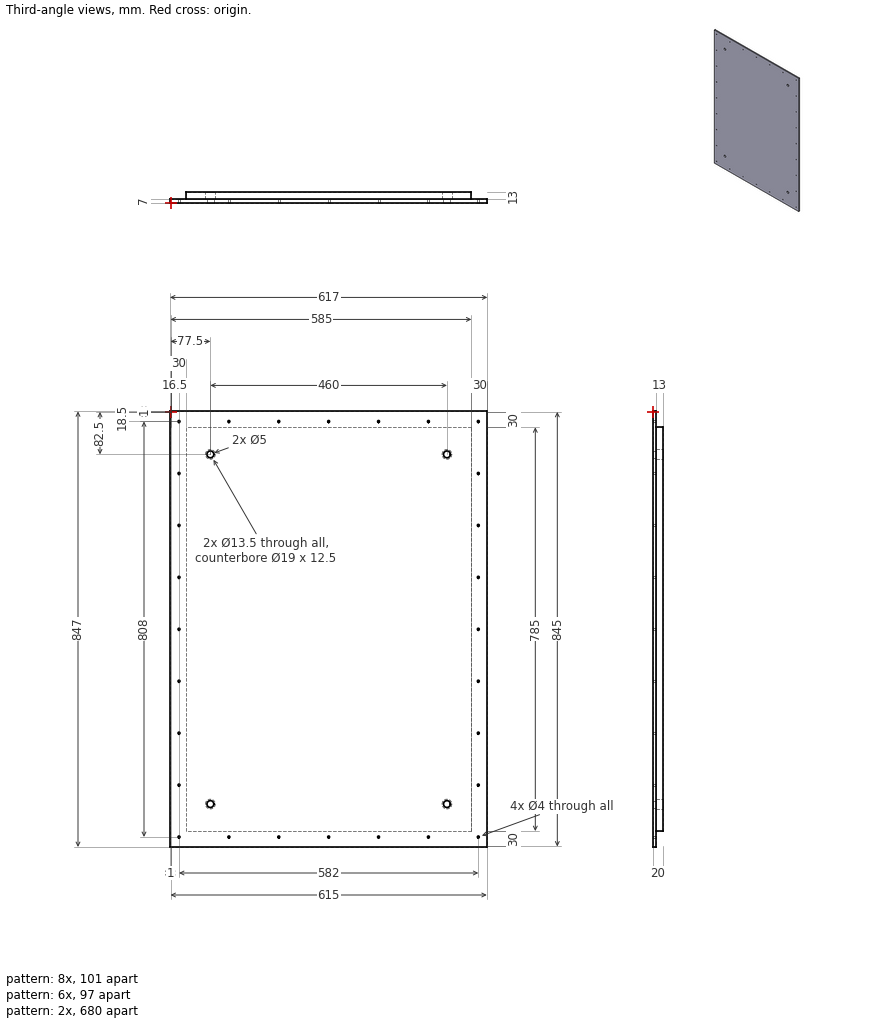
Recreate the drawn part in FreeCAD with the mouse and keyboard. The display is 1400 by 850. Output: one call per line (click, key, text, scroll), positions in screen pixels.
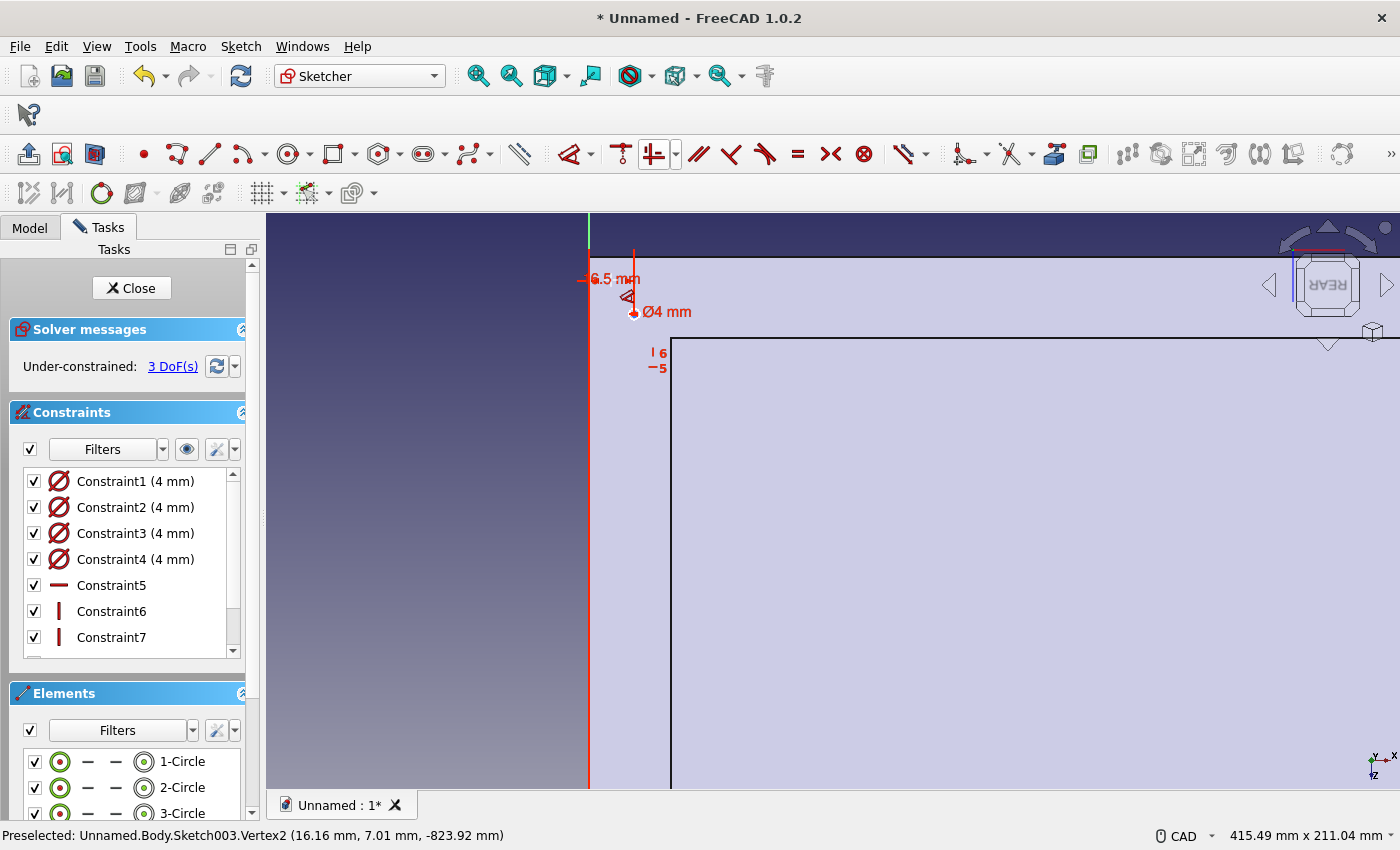
scroll(637, 317, down, 9)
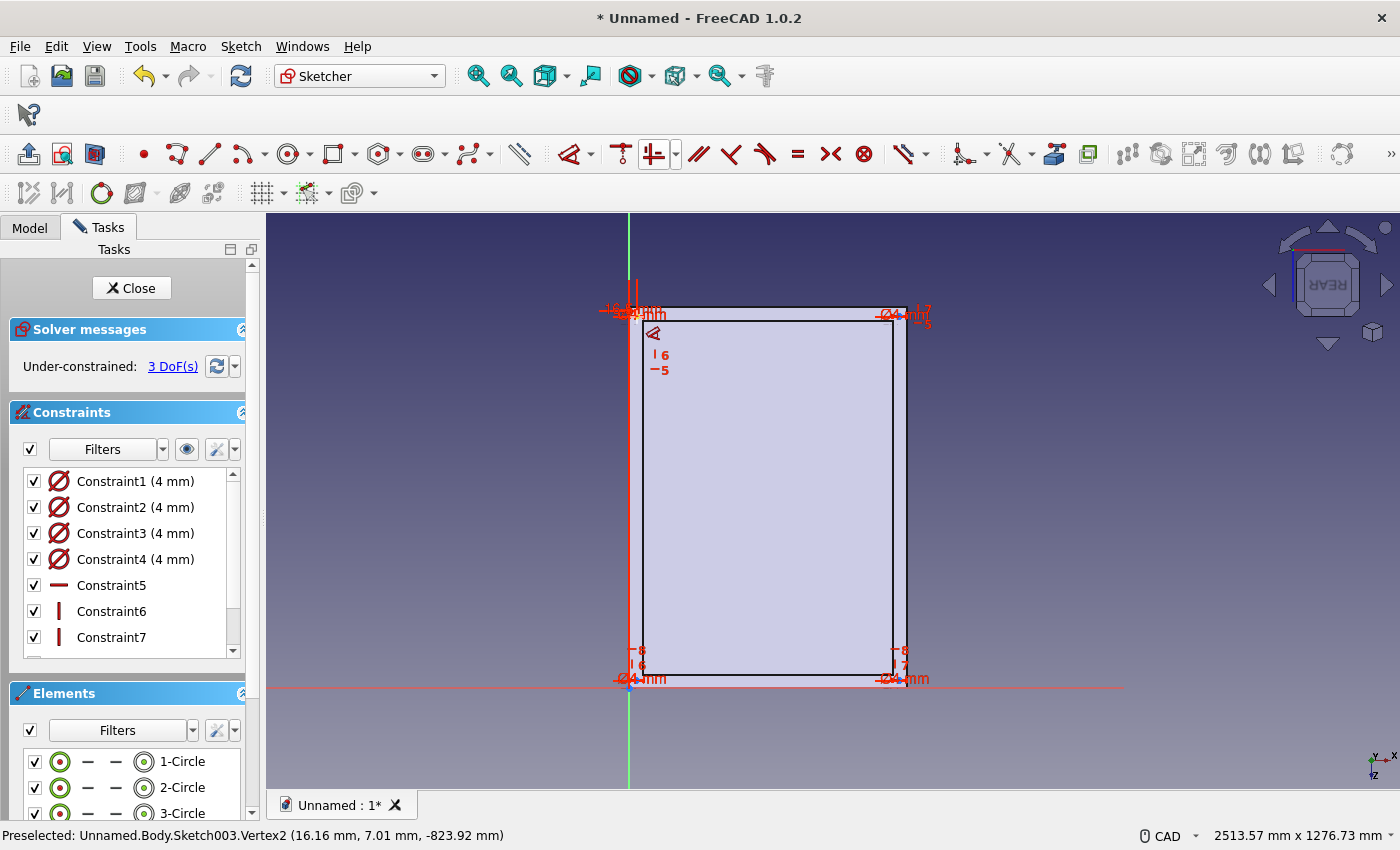
scroll(637, 681, up, 8)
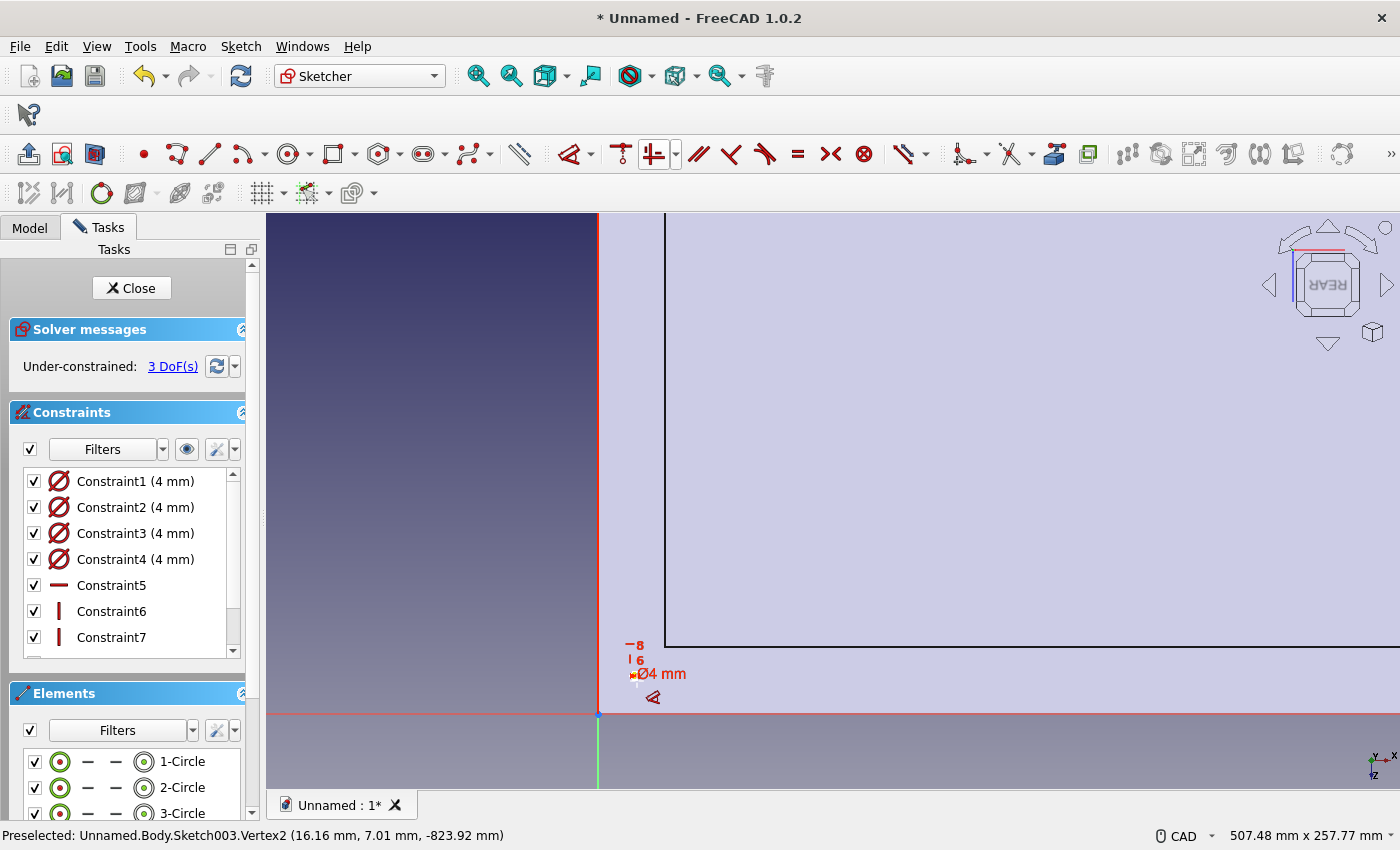
click(635, 676)
click(564, 695)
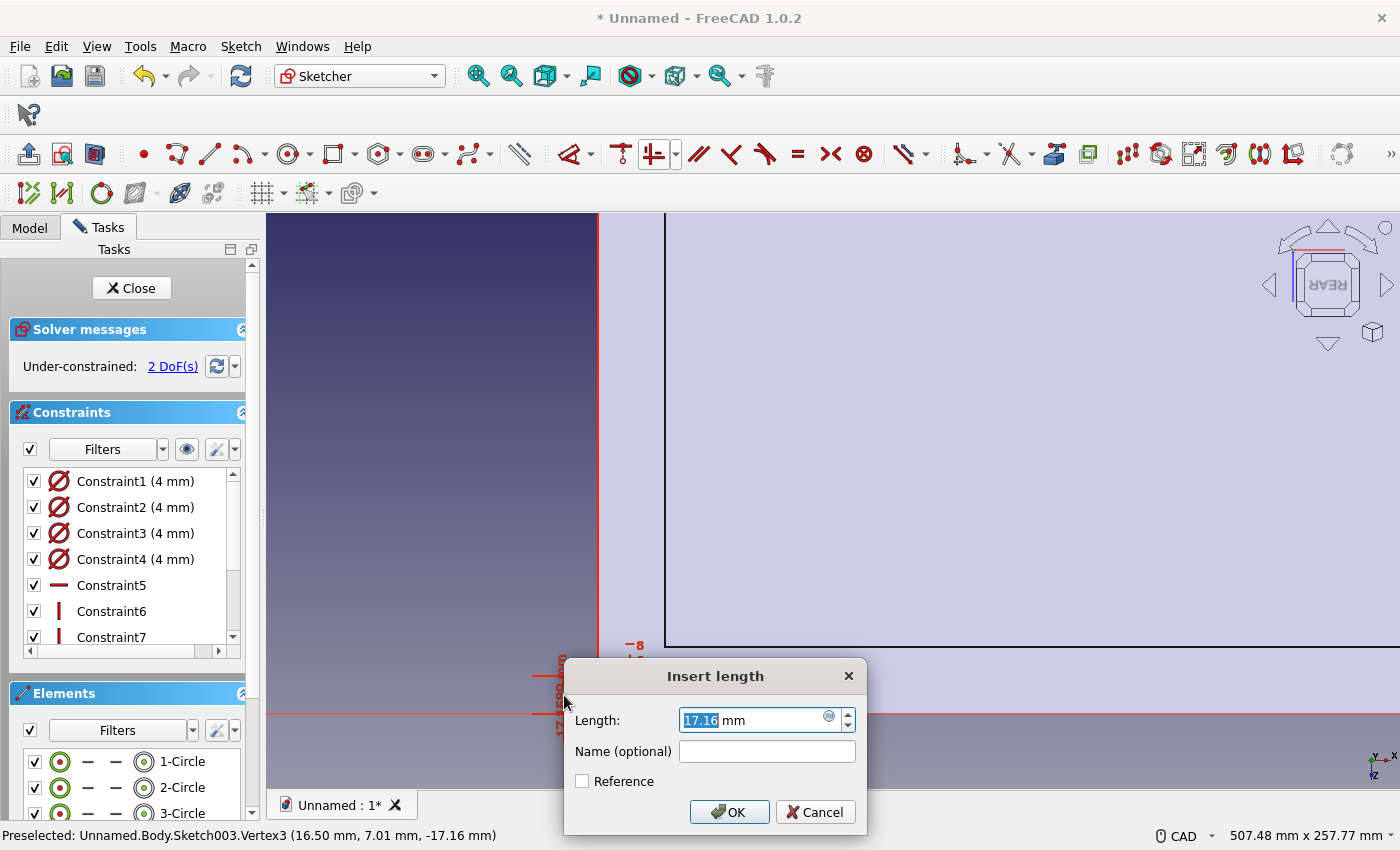
text(18.5)
key(Return)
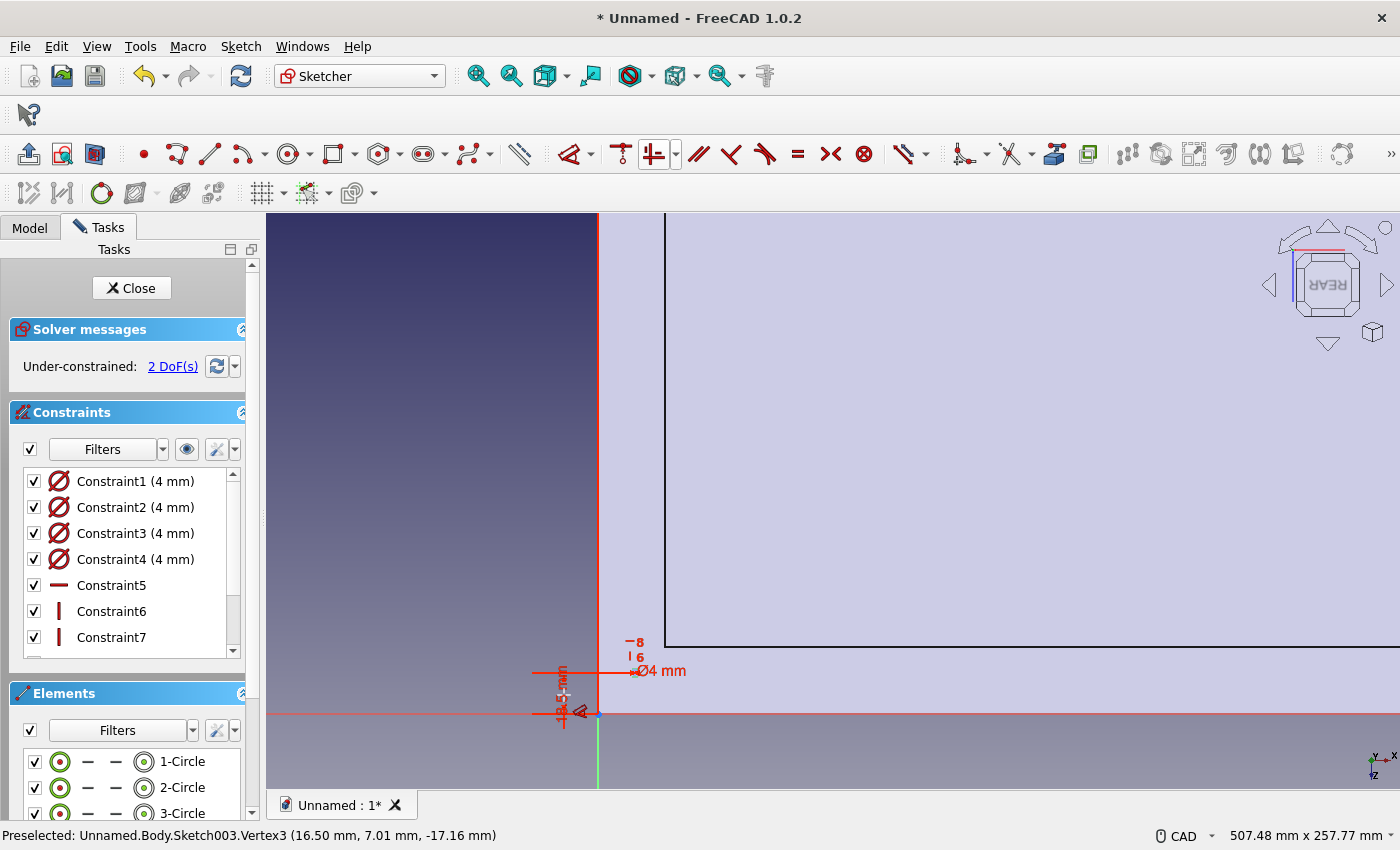
scroll(637, 681, down, 8)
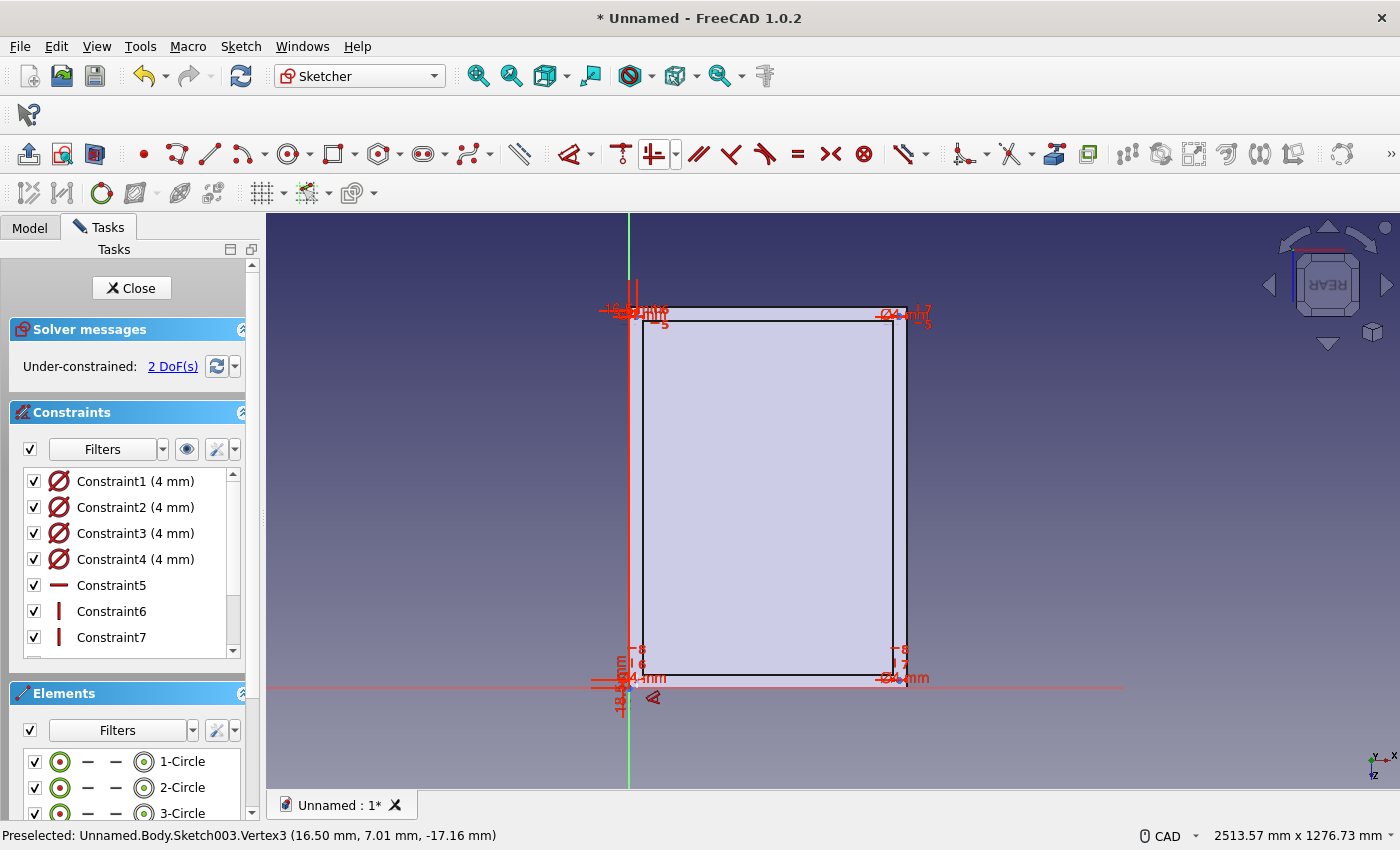
click(899, 317)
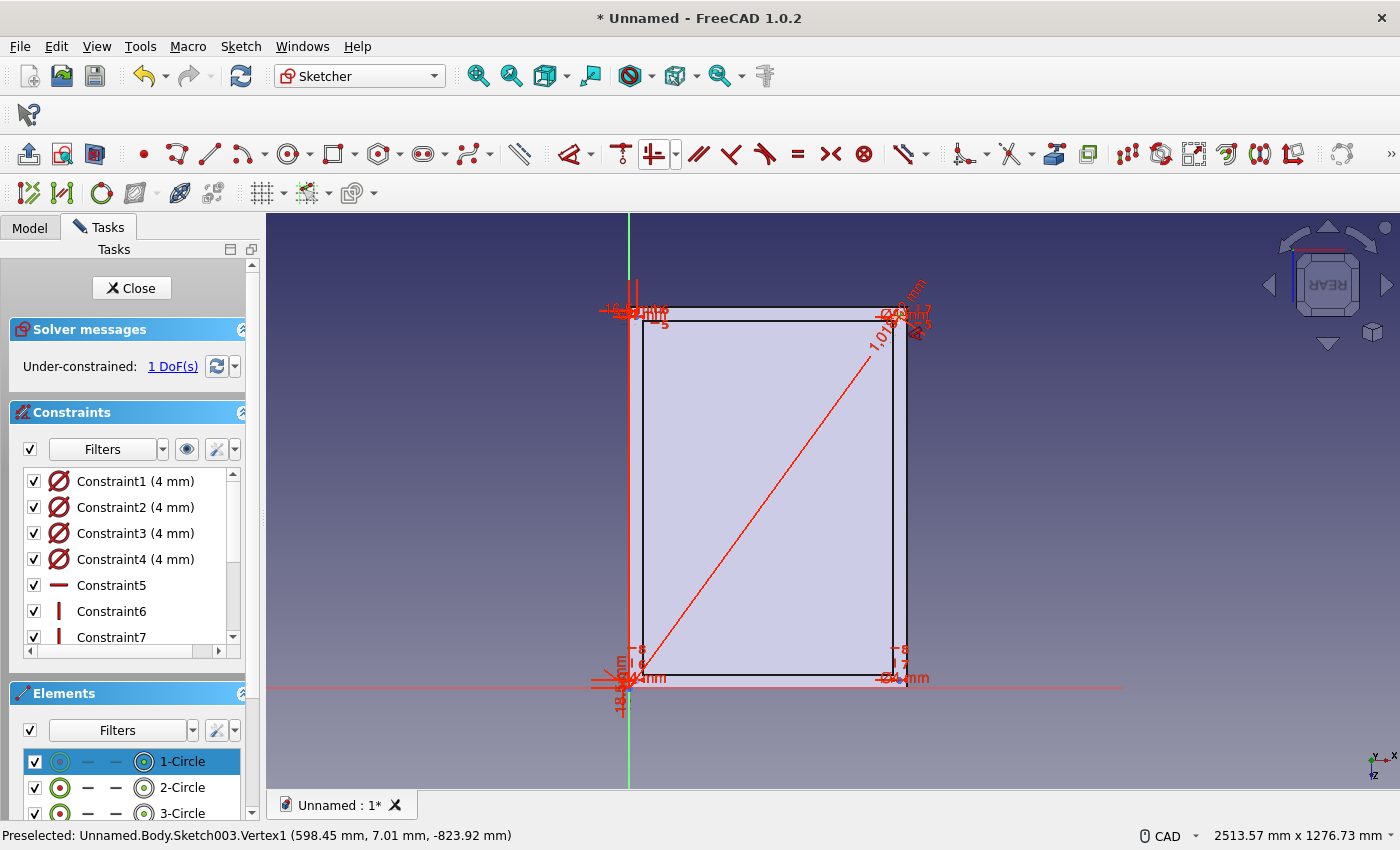
click(637, 317)
click(768, 283)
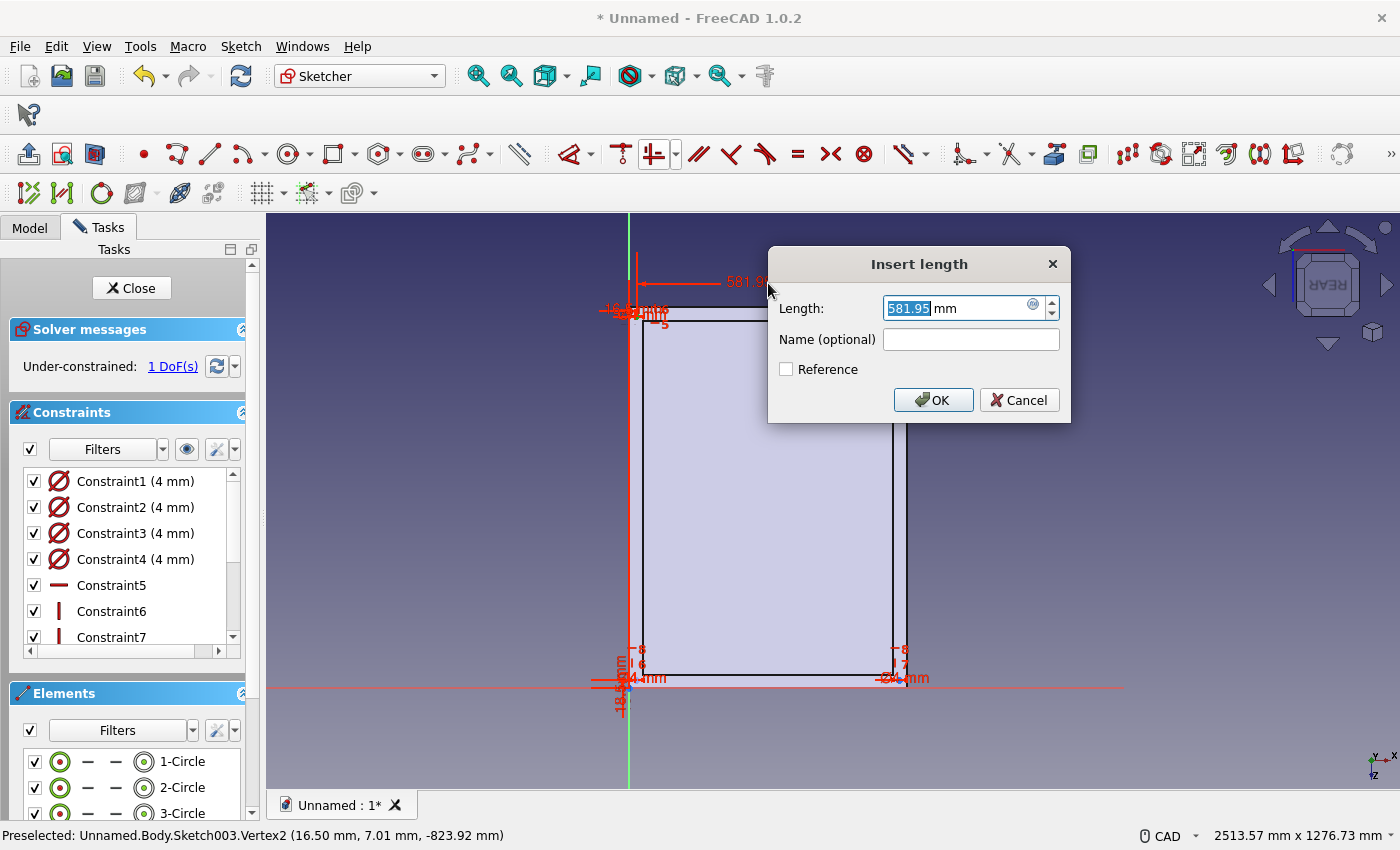
text(582)
key(Return)